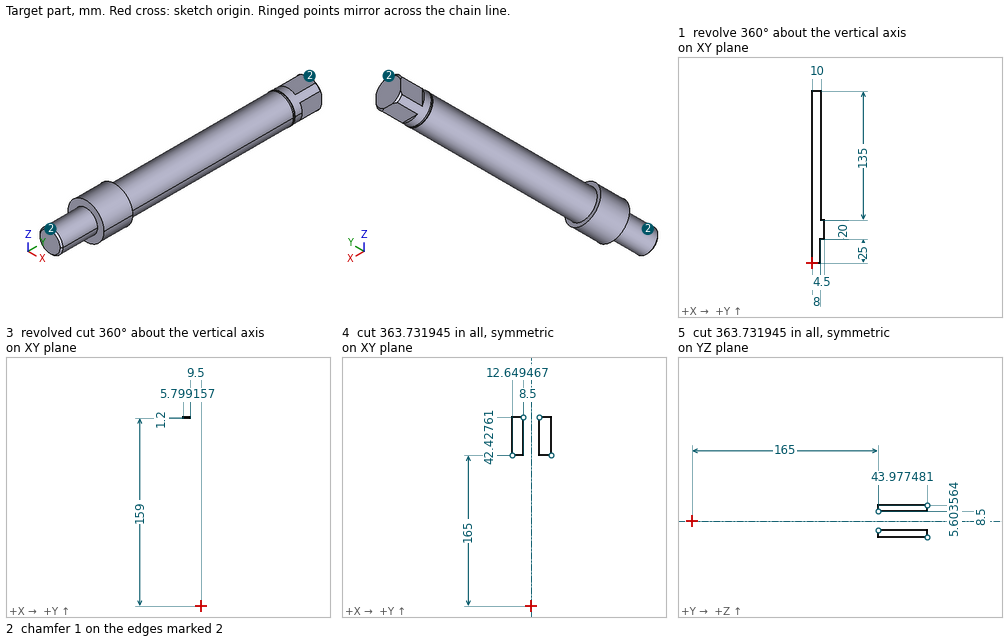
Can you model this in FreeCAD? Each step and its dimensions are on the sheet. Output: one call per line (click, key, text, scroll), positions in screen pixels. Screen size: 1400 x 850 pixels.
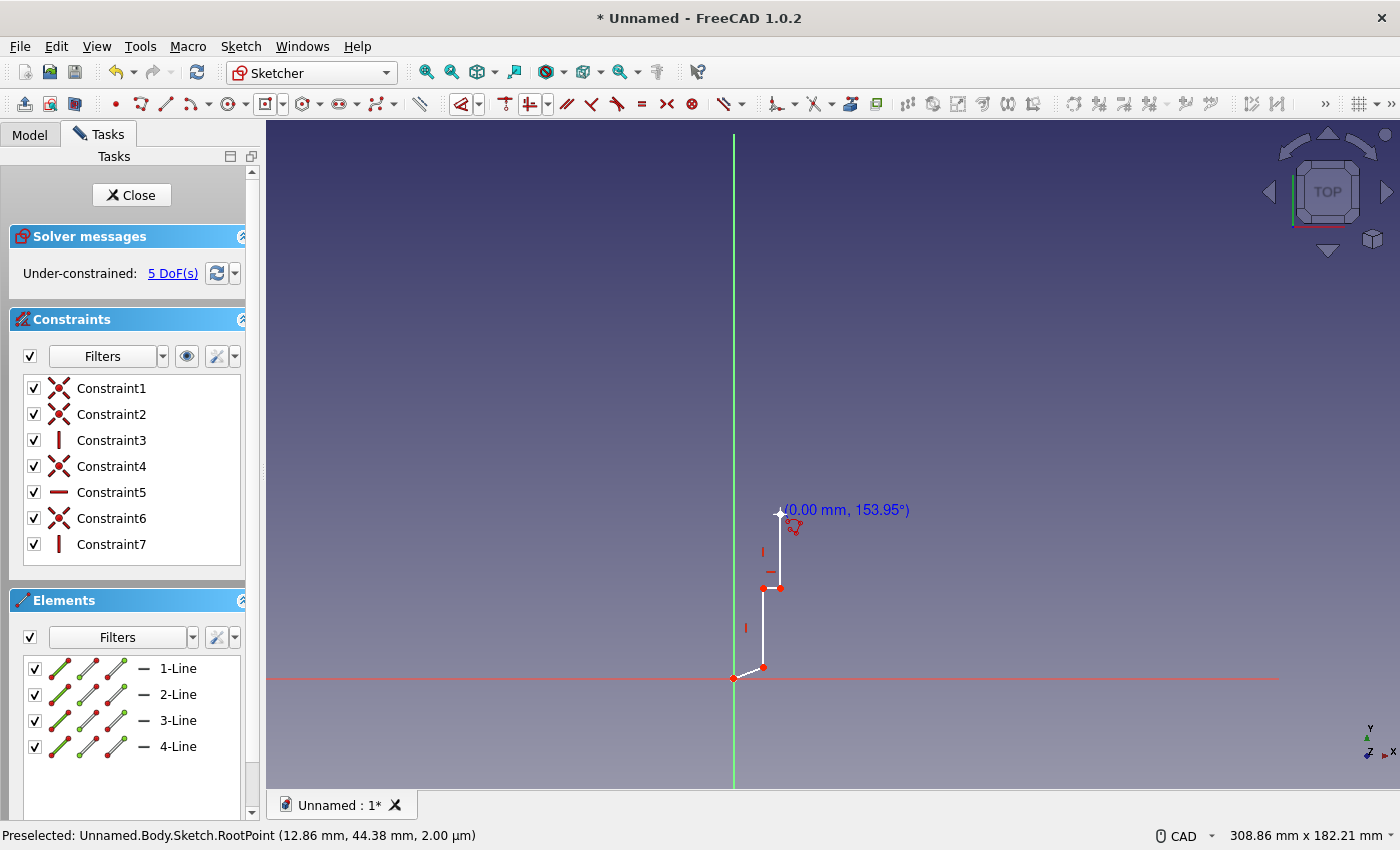
scroll(770, 514, up, 3)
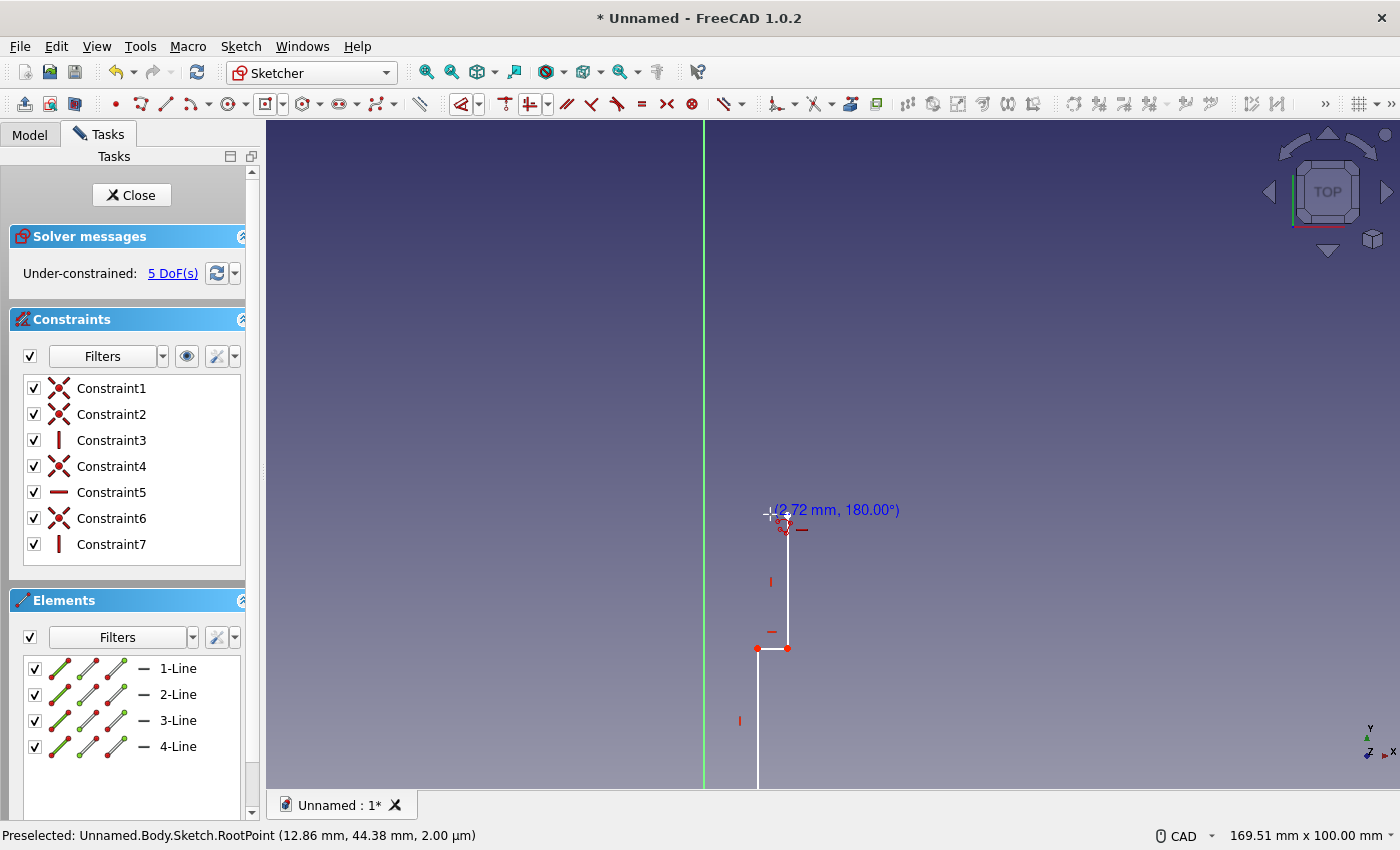
click(771, 514)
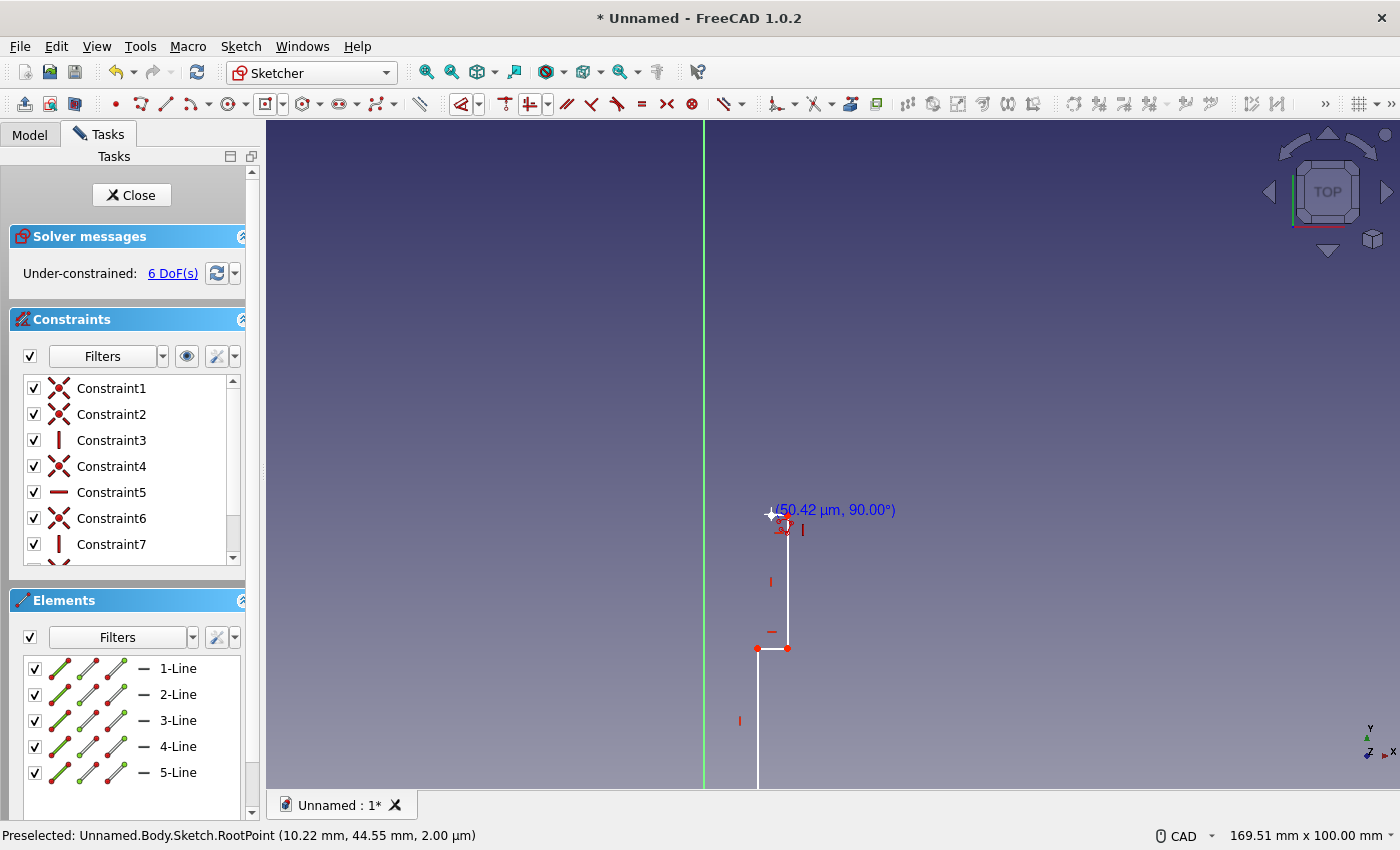
scroll(776, 596, down, 5)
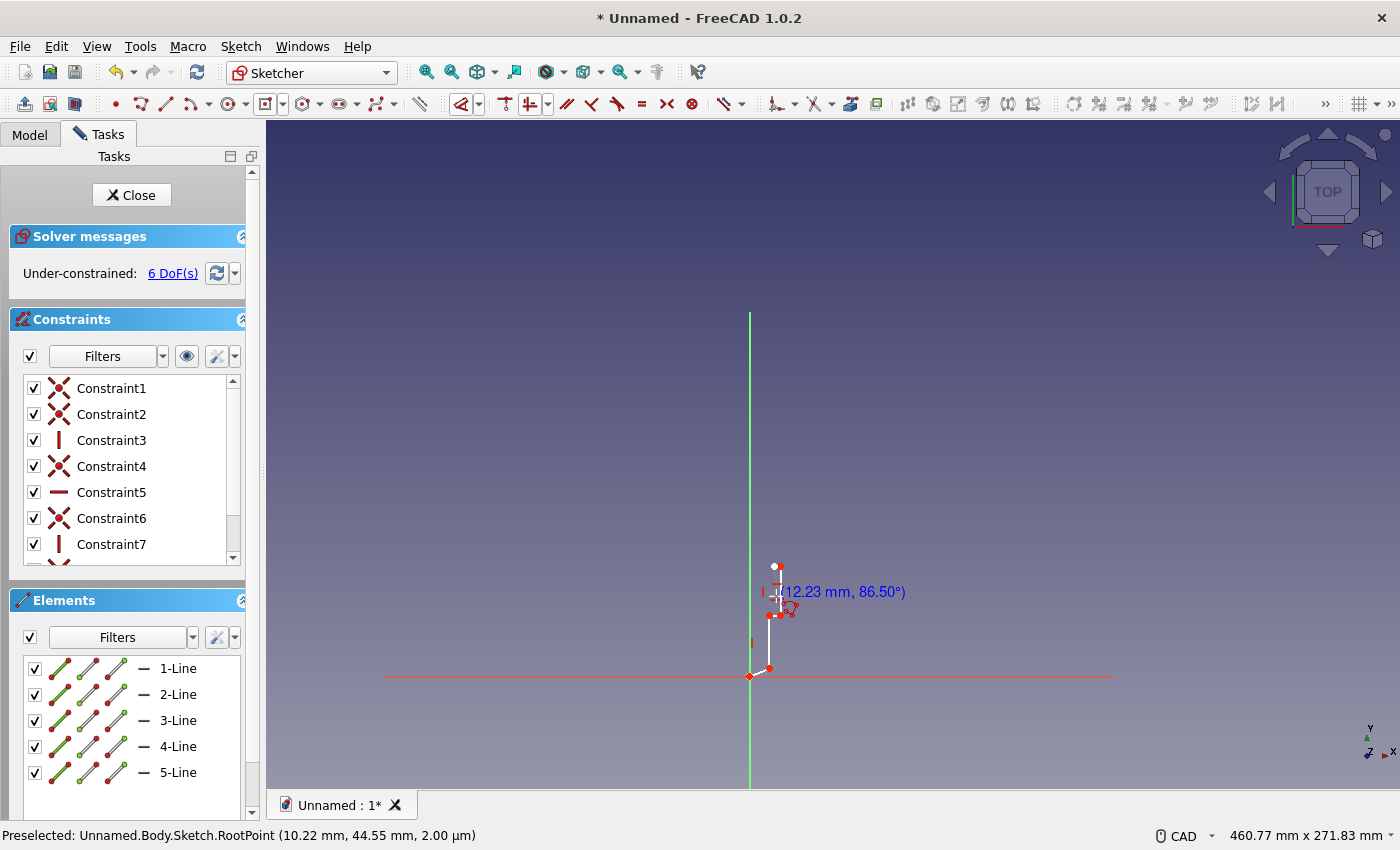
click(774, 234)
click(759, 234)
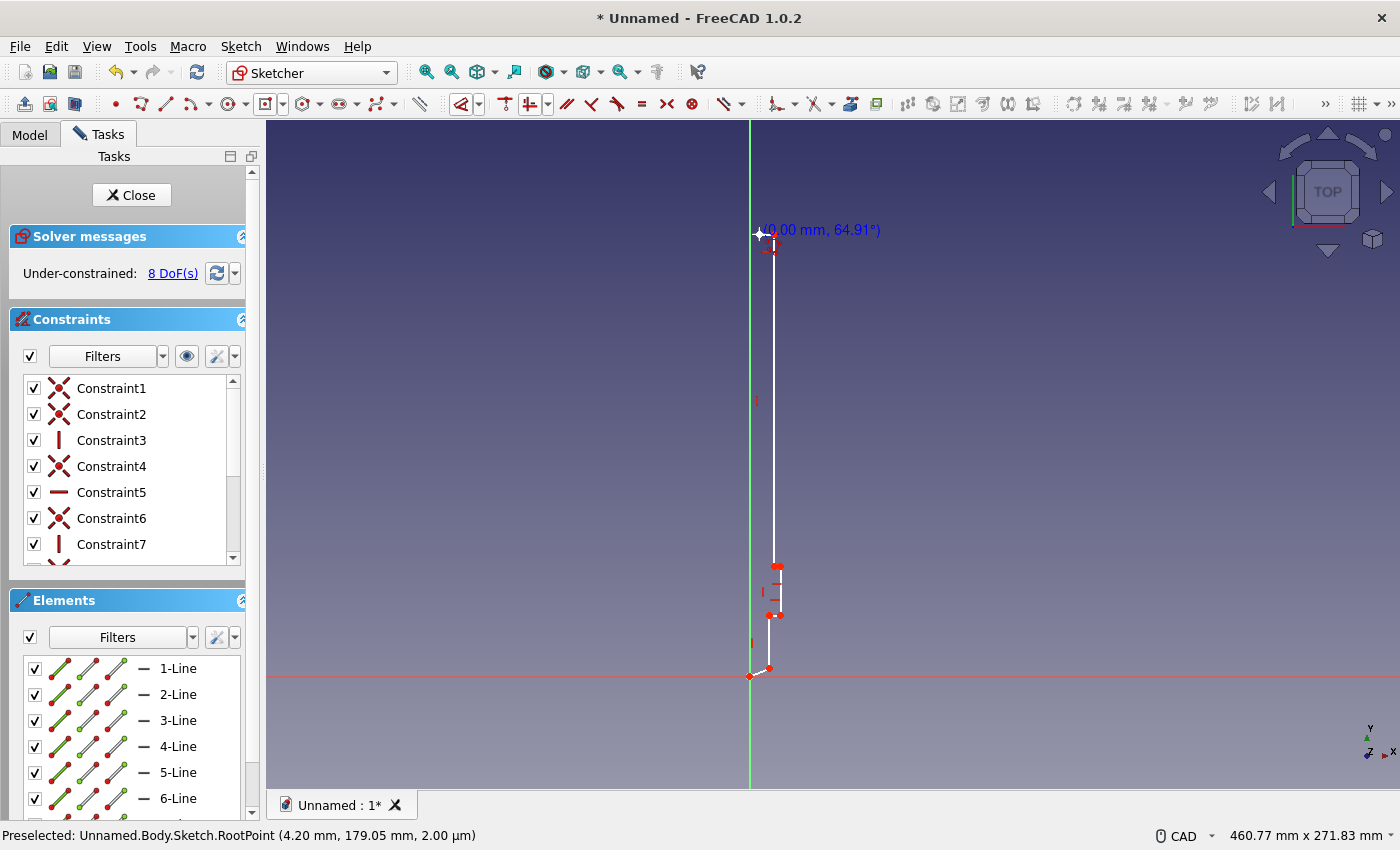
scroll(750, 677, up, 3)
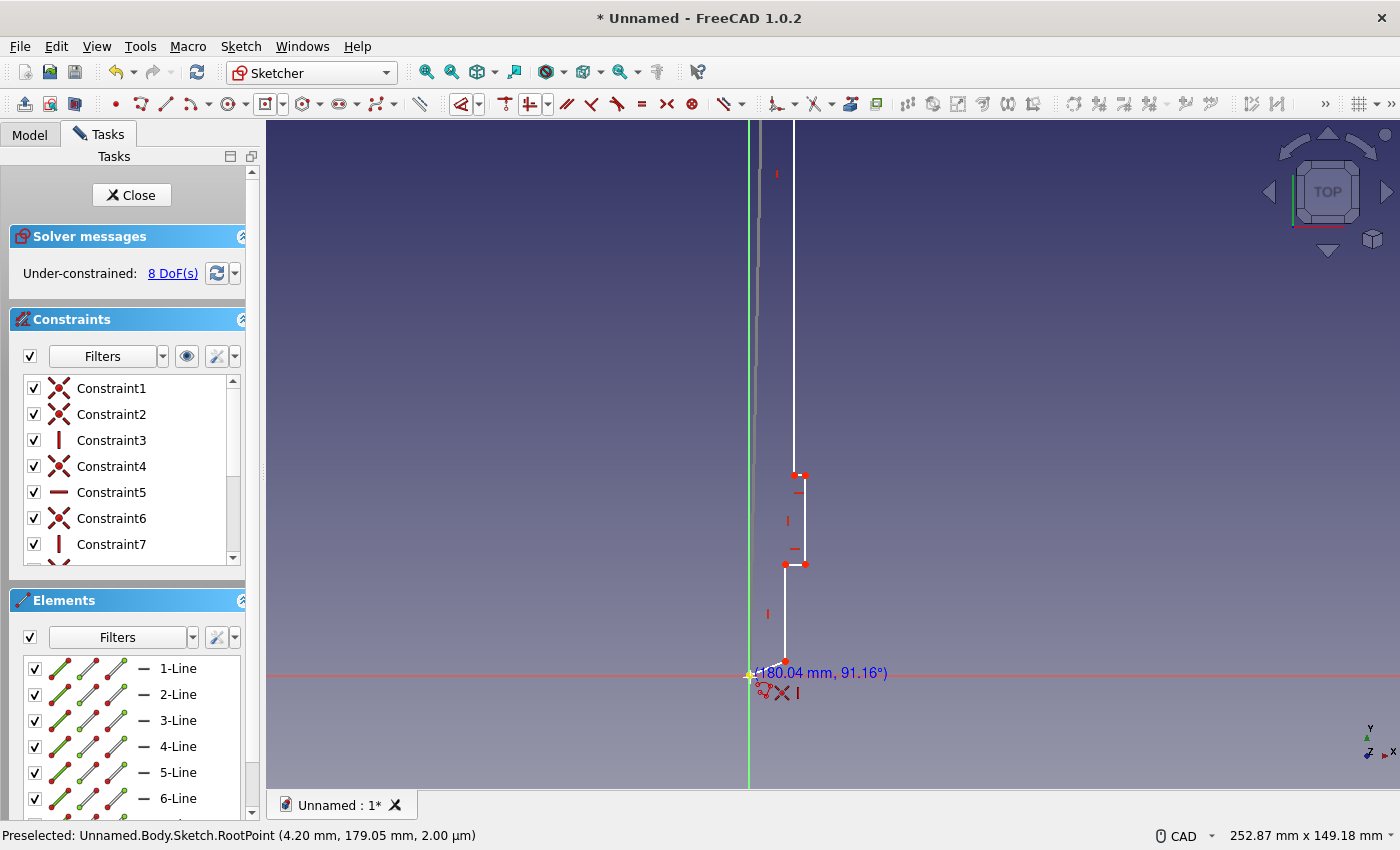
click(749, 676)
key(Escape)
key(Escape)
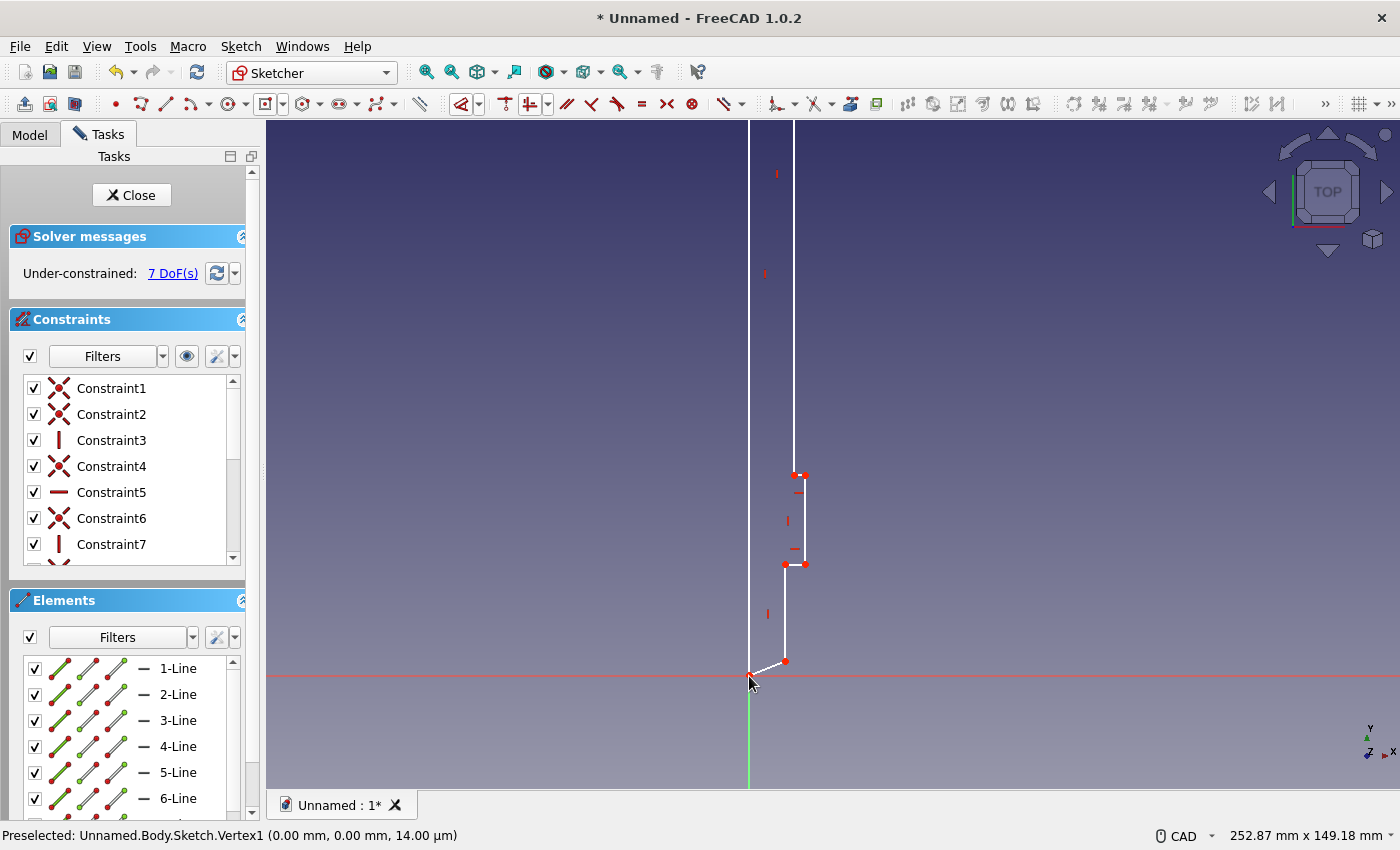
scroll(774, 666, up, 2)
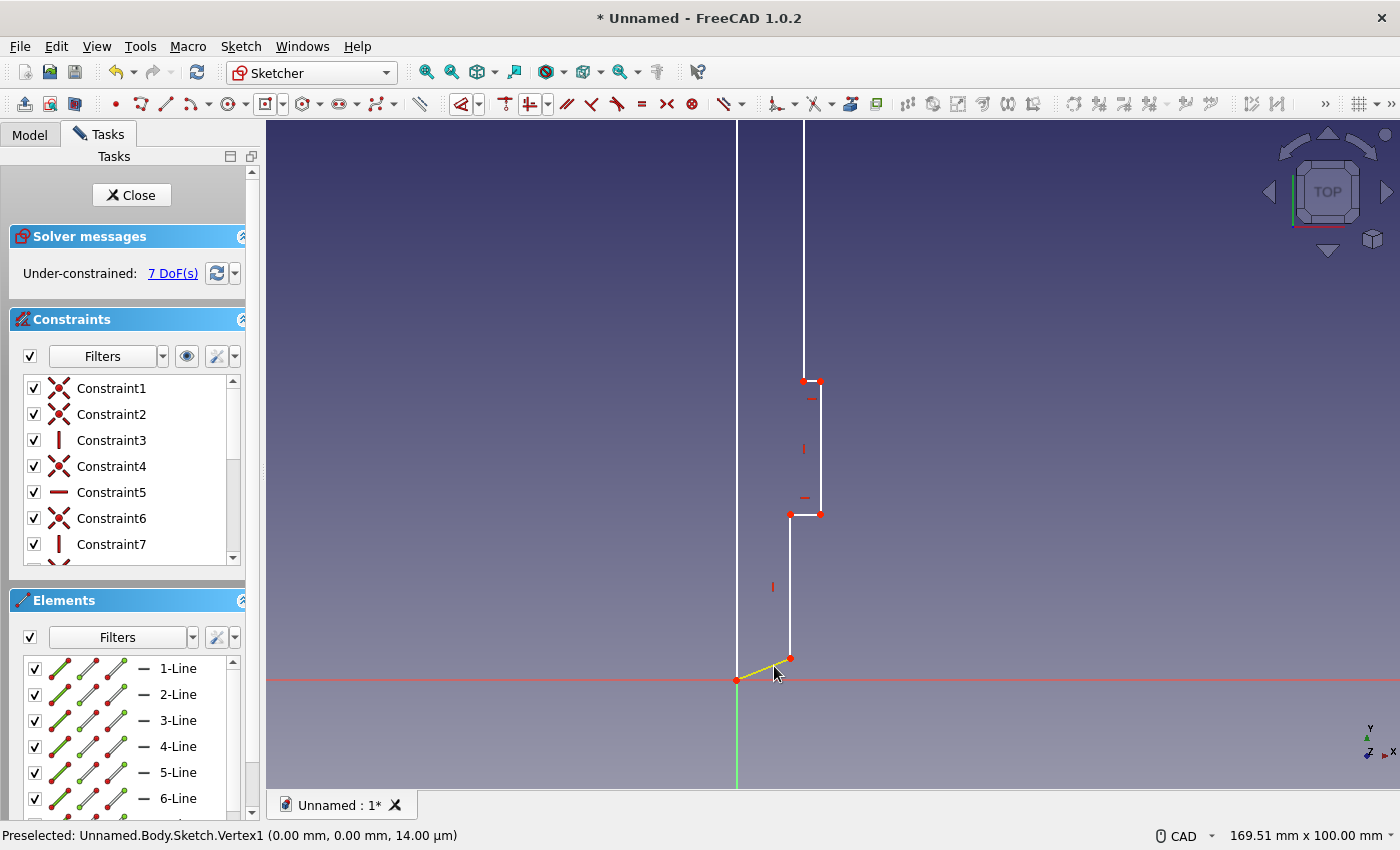
click(774, 665)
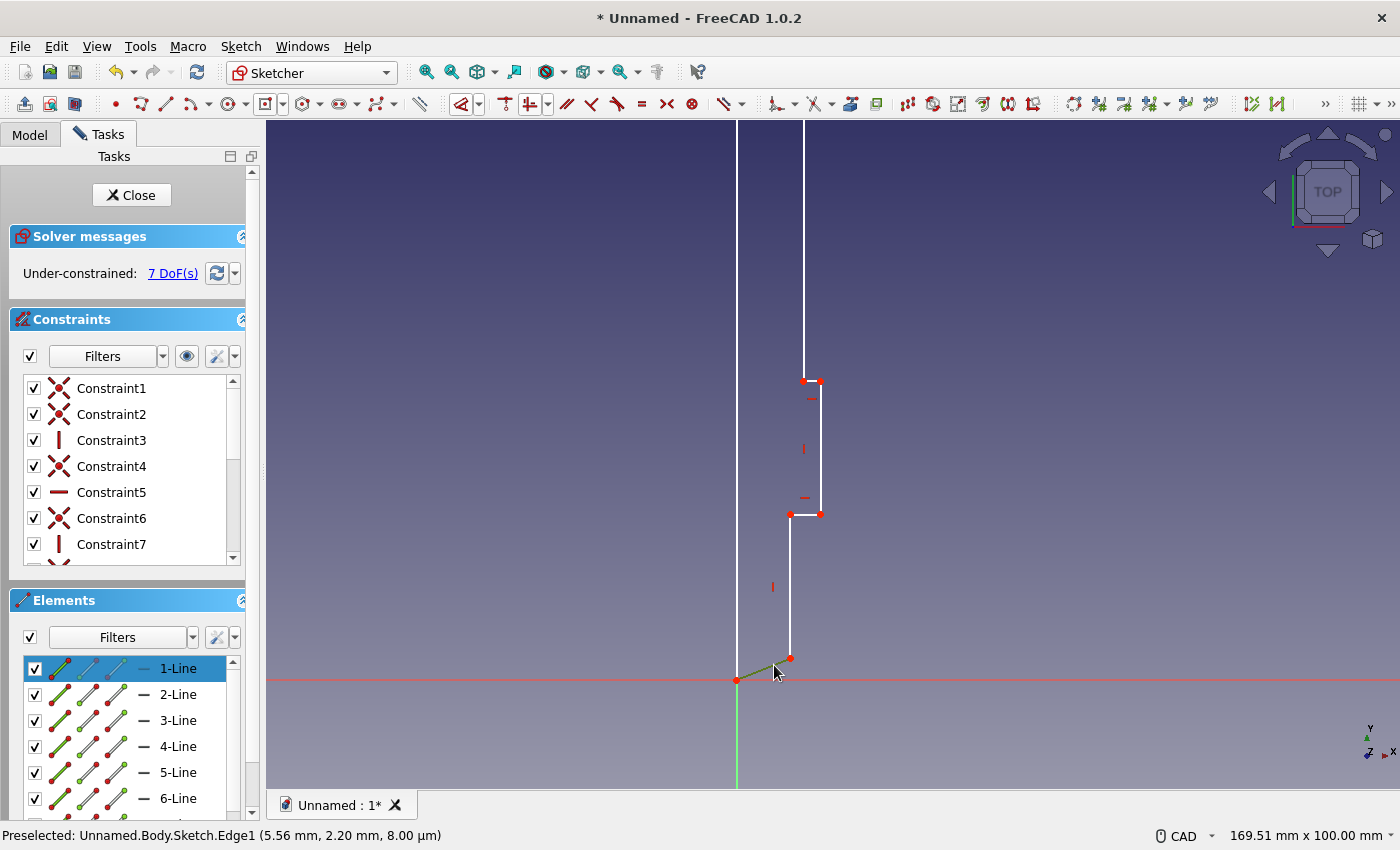
click(548, 104)